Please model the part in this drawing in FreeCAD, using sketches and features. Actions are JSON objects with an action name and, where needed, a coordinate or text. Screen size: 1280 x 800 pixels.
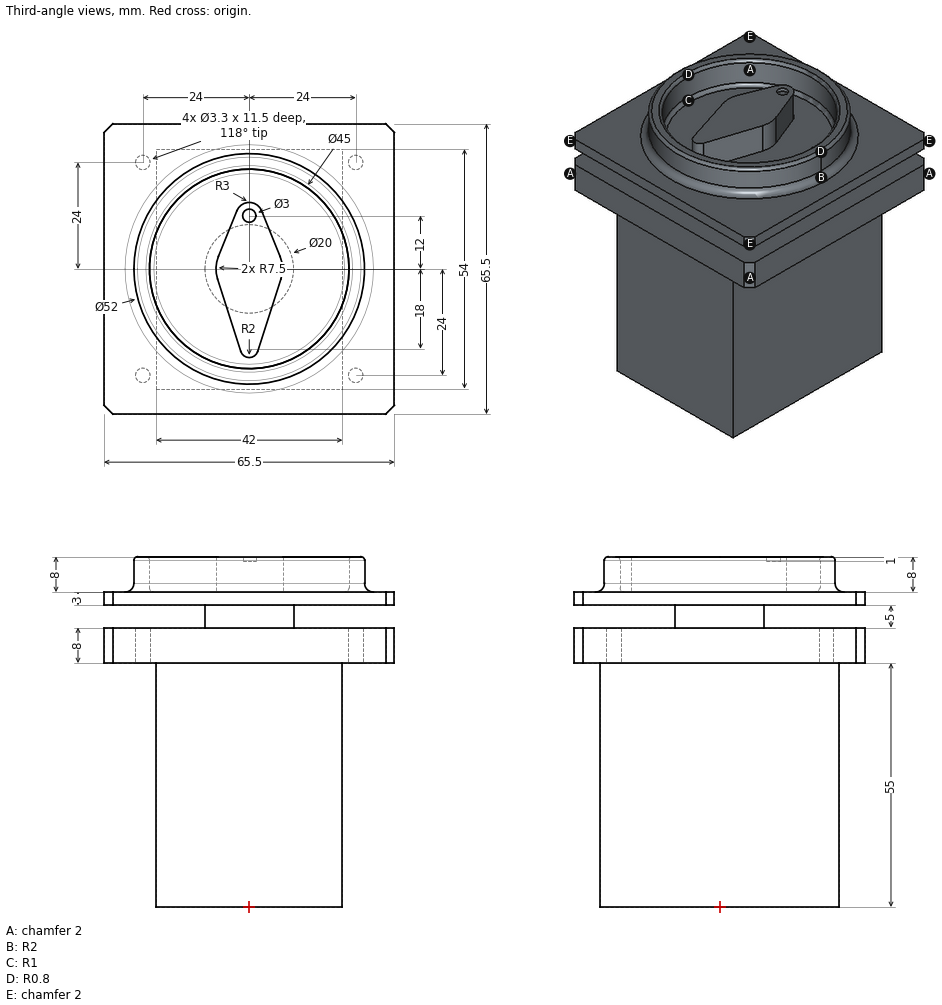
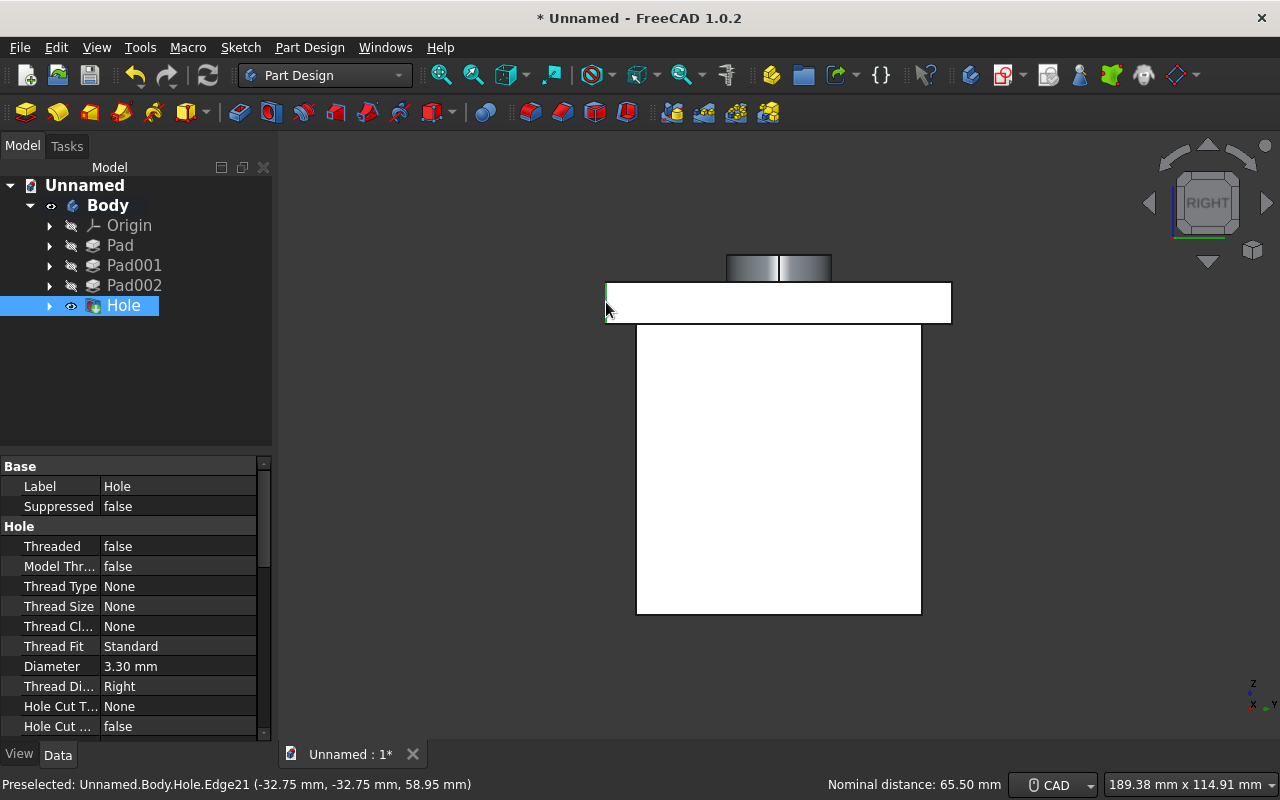
{"action": "left_click", "coordinate": [952, 302], "text": "ctrl"}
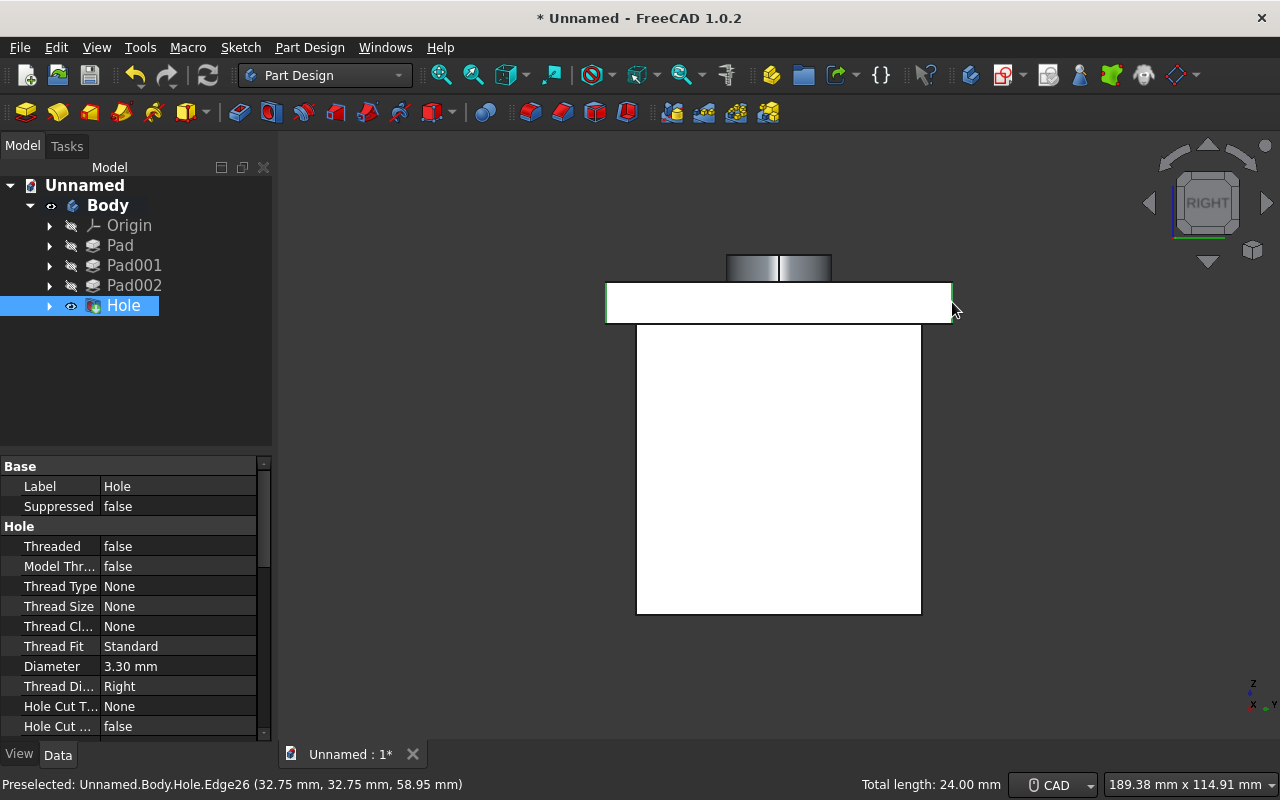
{"action": "key", "text": "5"}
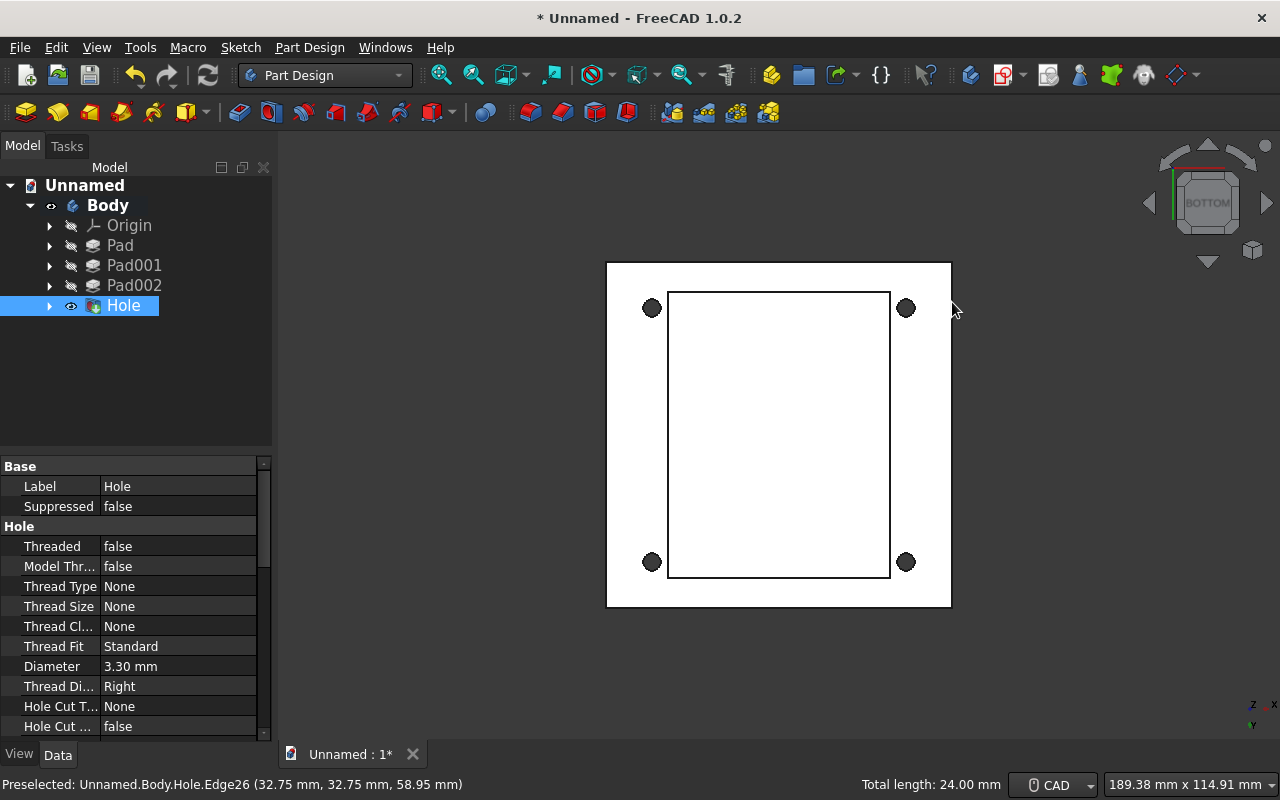
{"action": "key", "text": "4"}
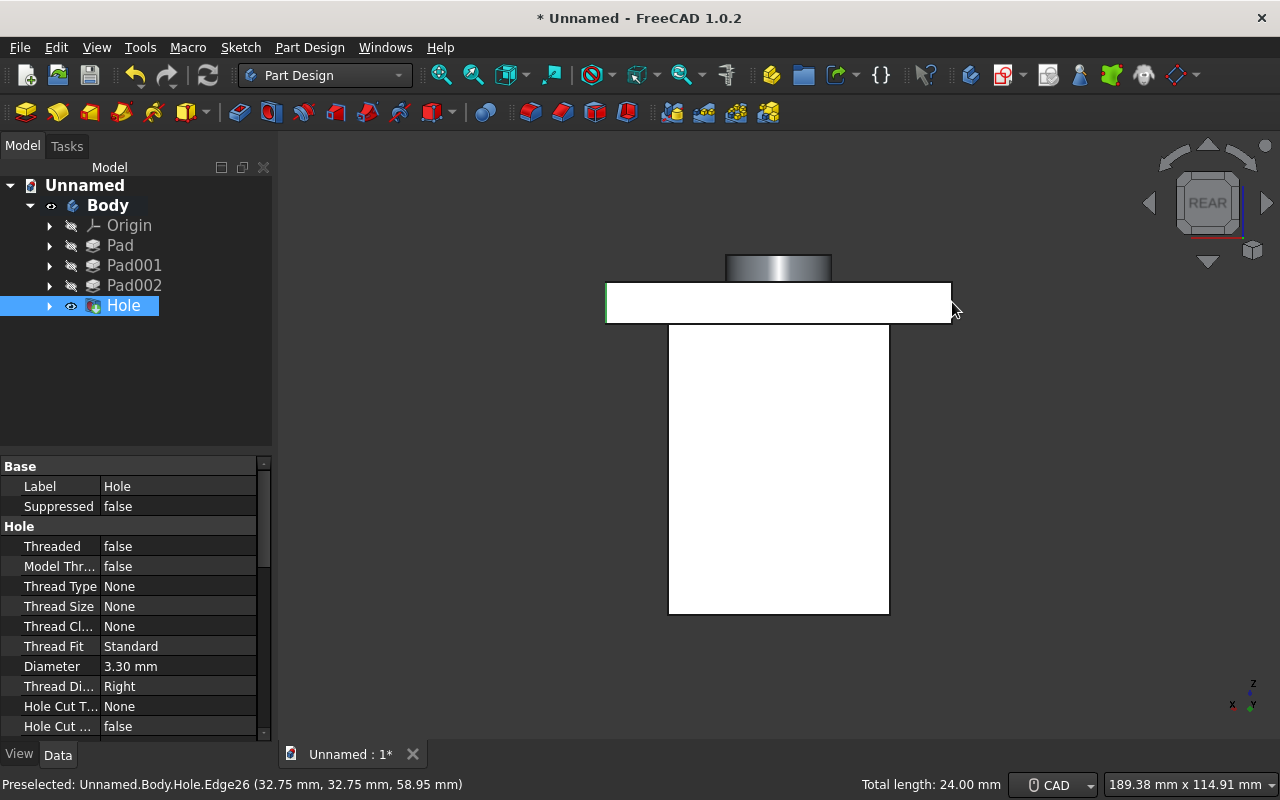
{"action": "left_click", "coordinate": [952, 302], "text": "ctrl"}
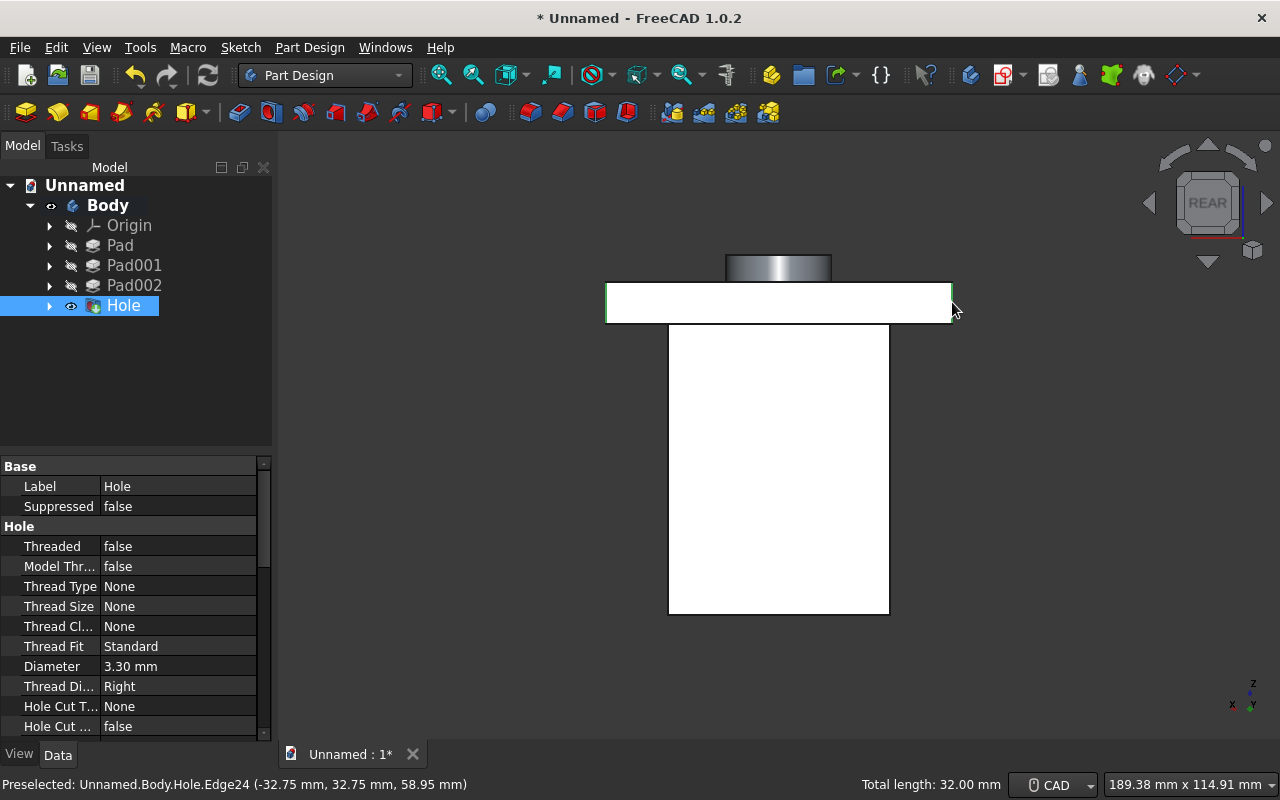
{"action": "left_click", "coordinate": [564, 112]}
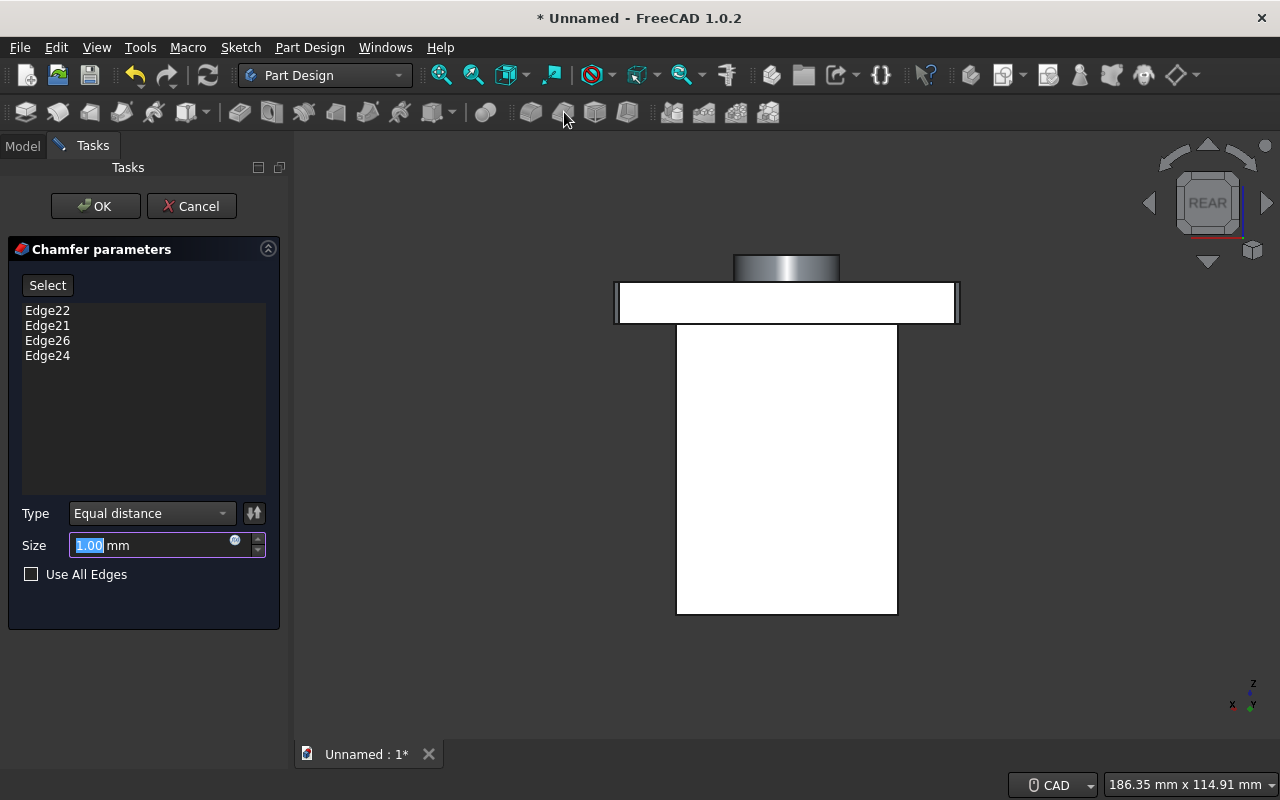
{"action": "type", "text": "2"}
{"action": "key", "text": "Tab"}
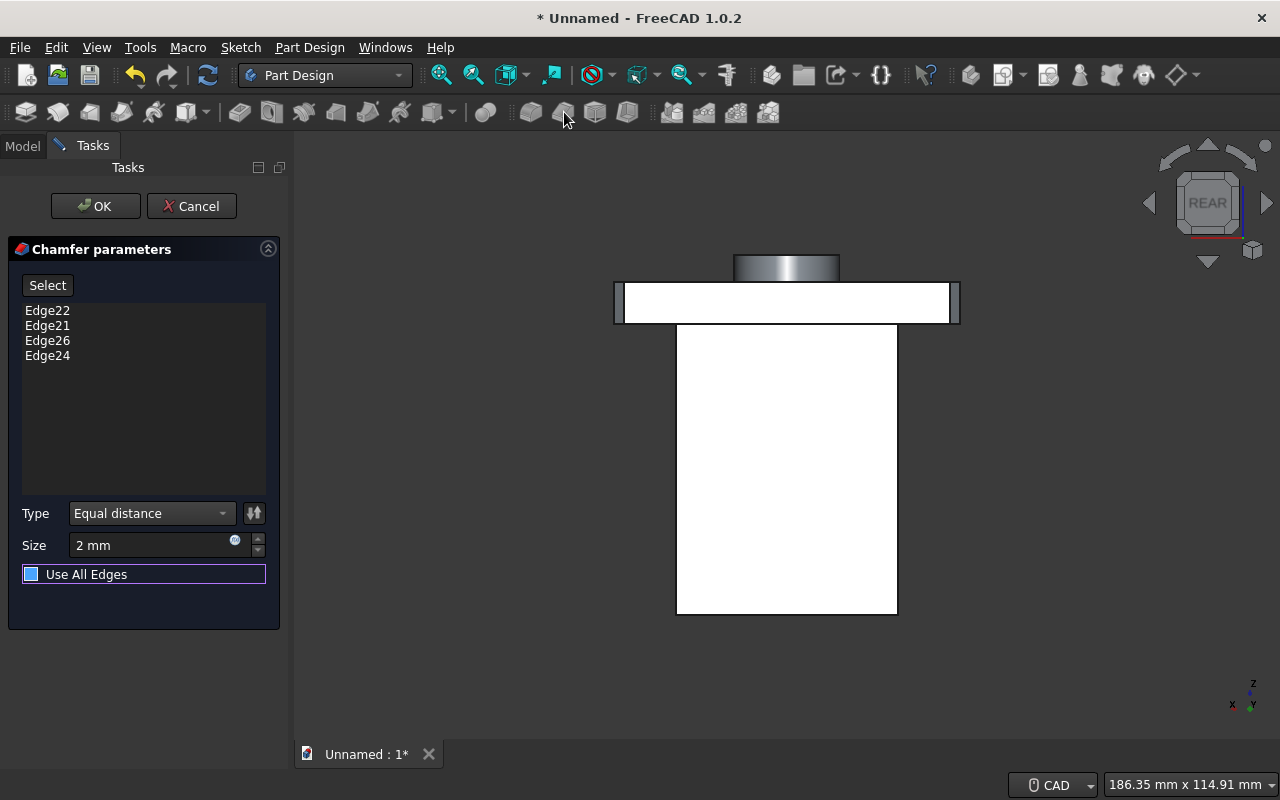
{"action": "left_click", "coordinate": [96, 206]}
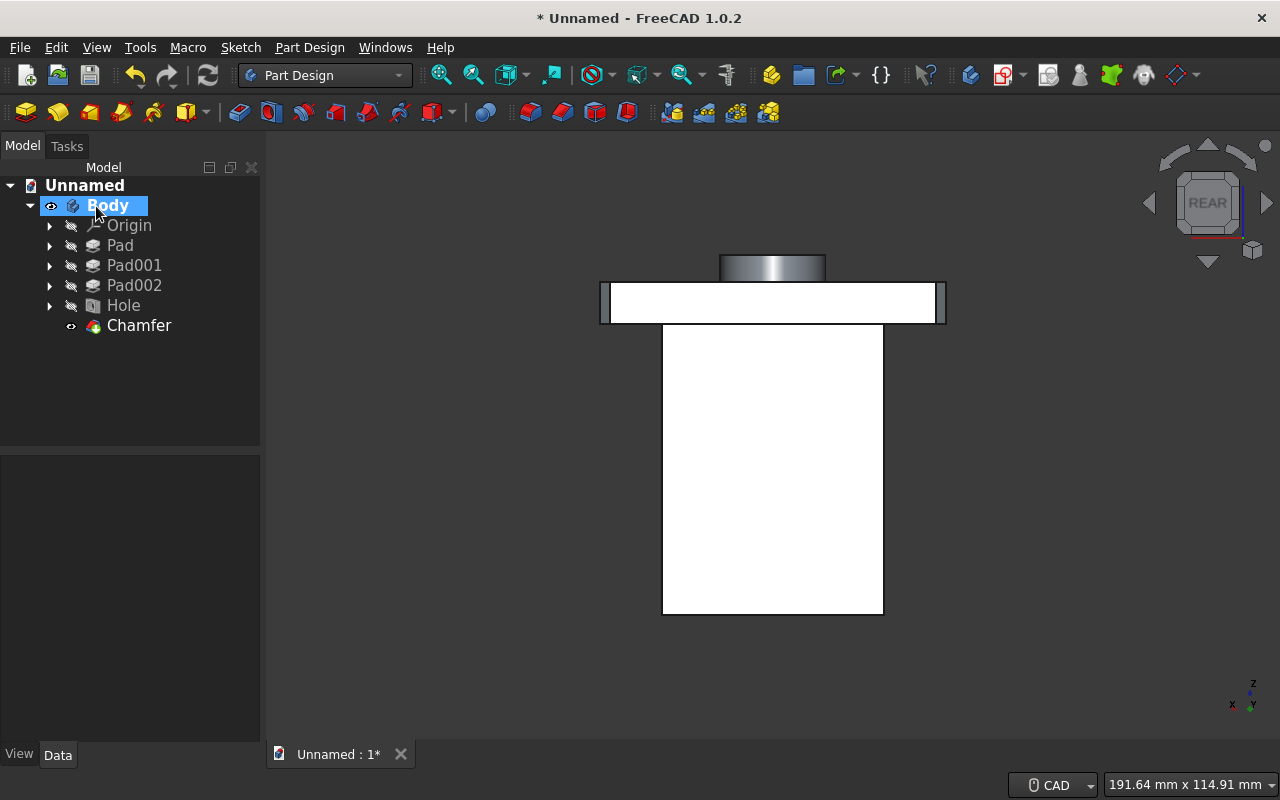
{"action": "key", "text": "0"}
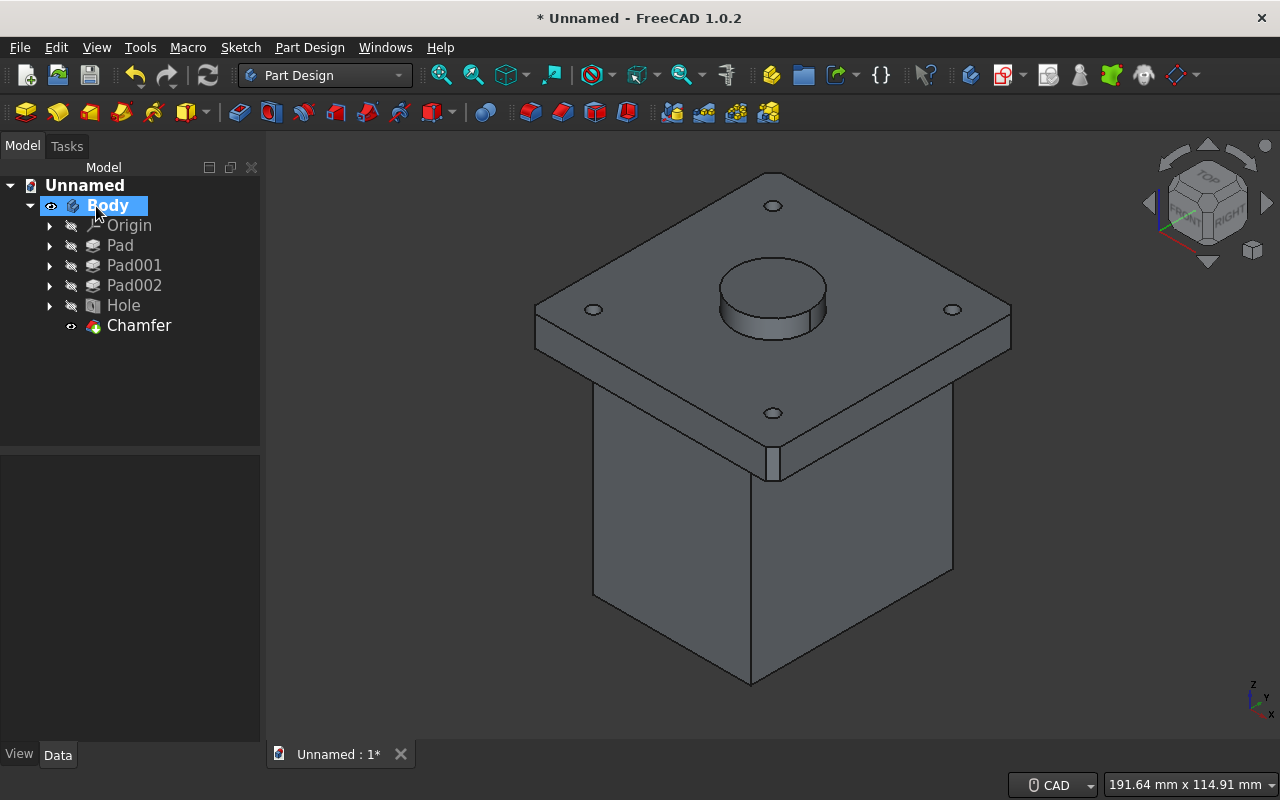
{"action": "left_click", "coordinate": [773, 287]}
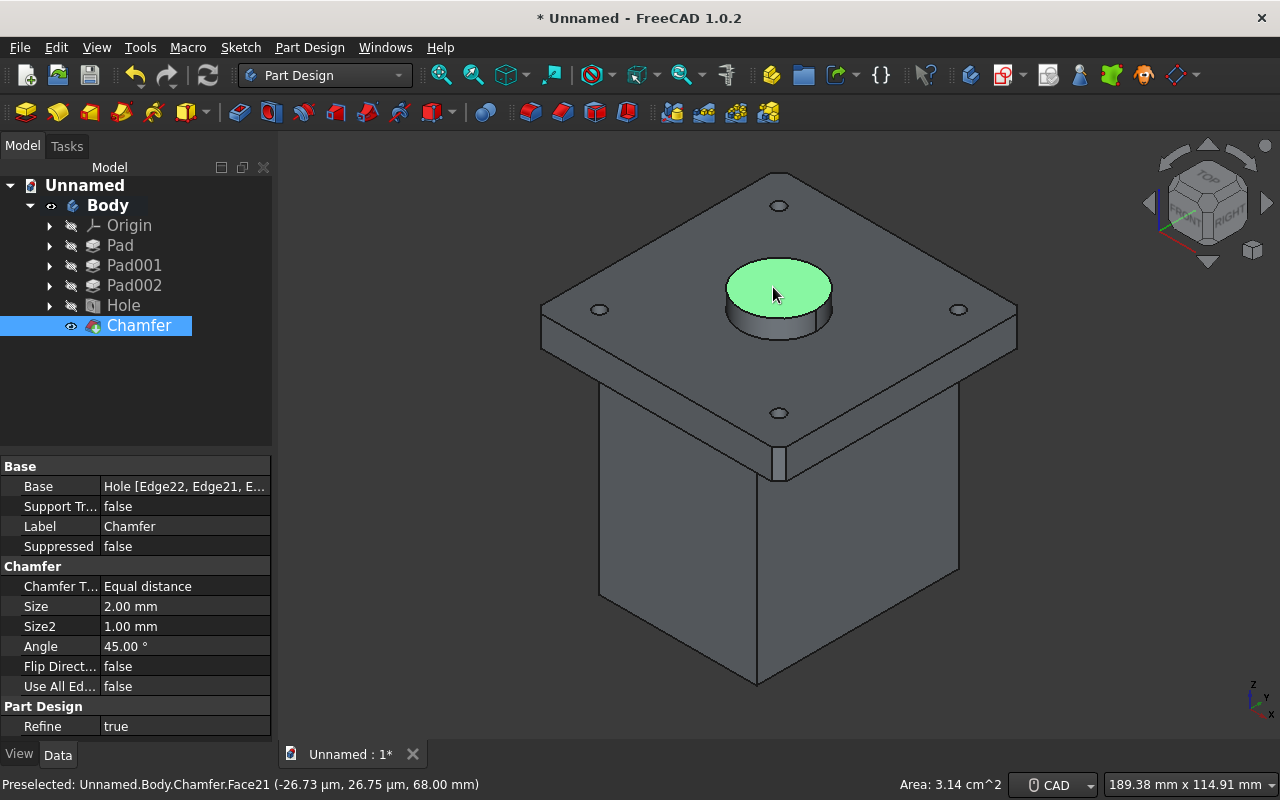
{"action": "left_click", "coordinate": [1004, 76]}